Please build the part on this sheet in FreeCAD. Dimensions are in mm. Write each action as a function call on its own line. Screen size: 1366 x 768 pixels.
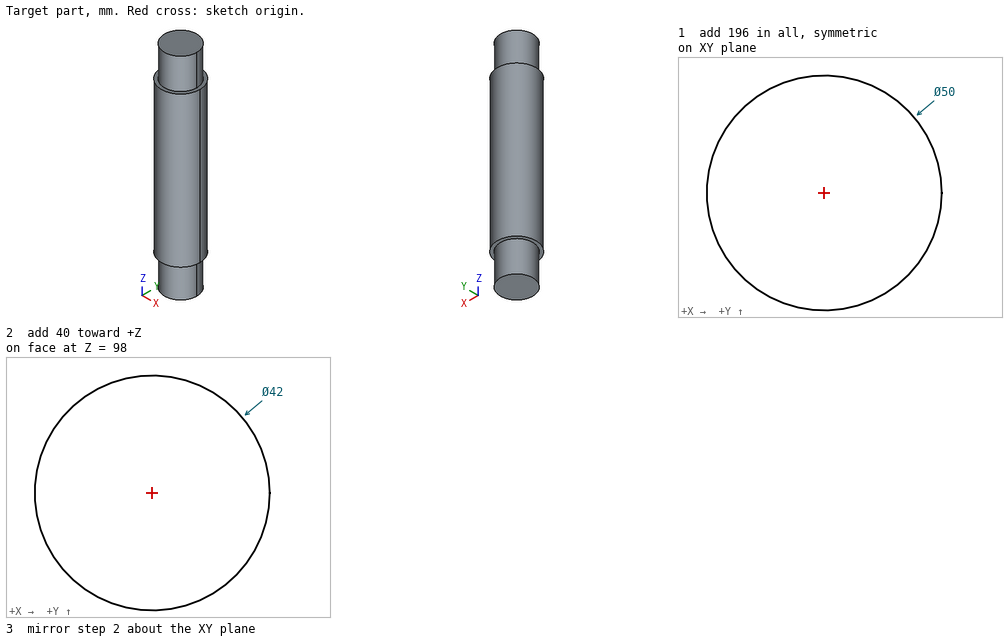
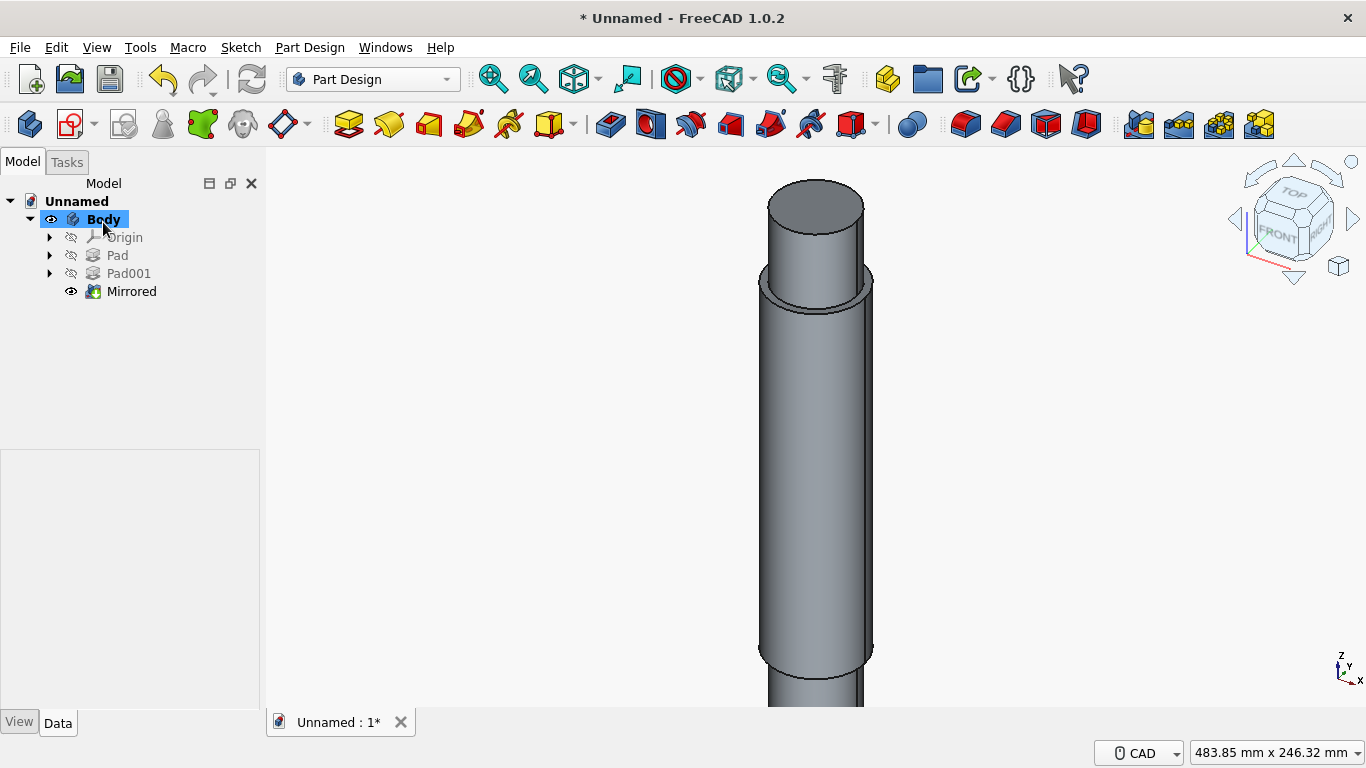
key(0)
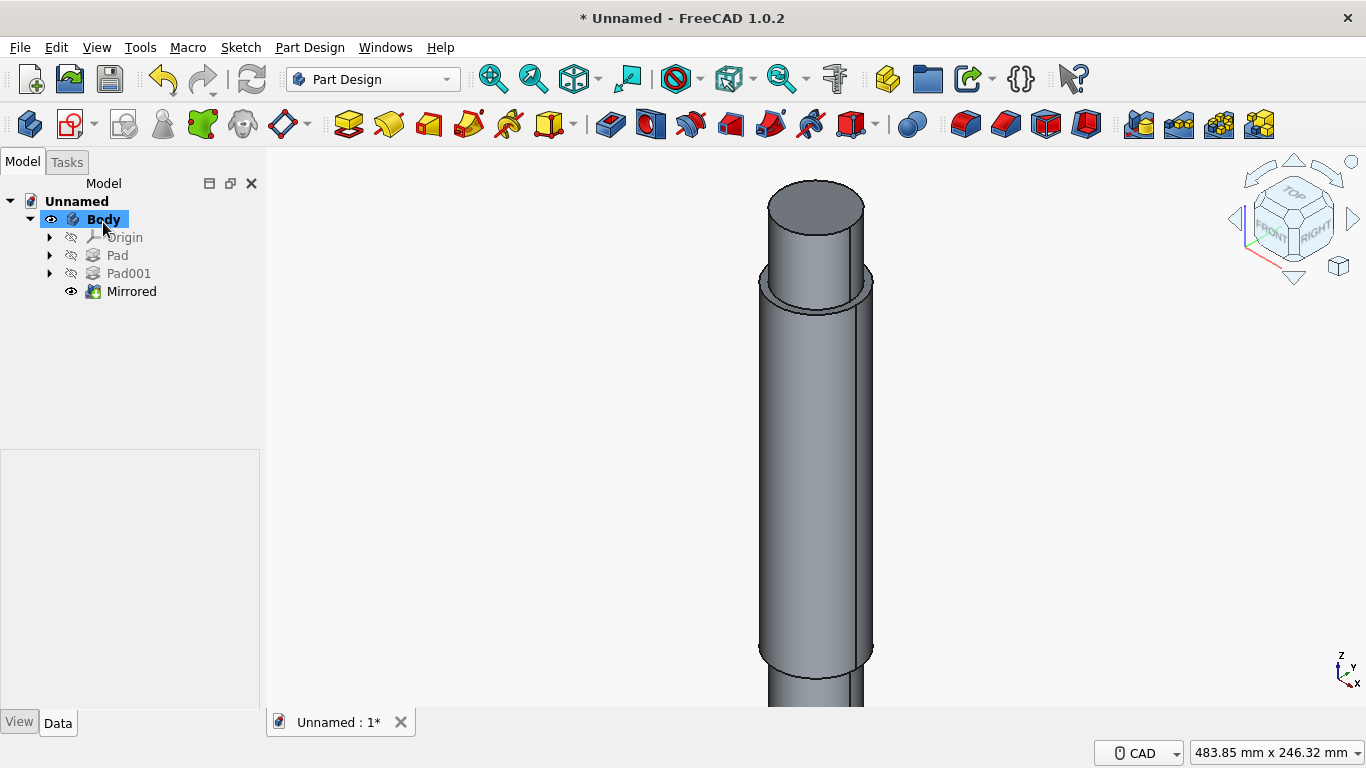
key(v)
key(f)